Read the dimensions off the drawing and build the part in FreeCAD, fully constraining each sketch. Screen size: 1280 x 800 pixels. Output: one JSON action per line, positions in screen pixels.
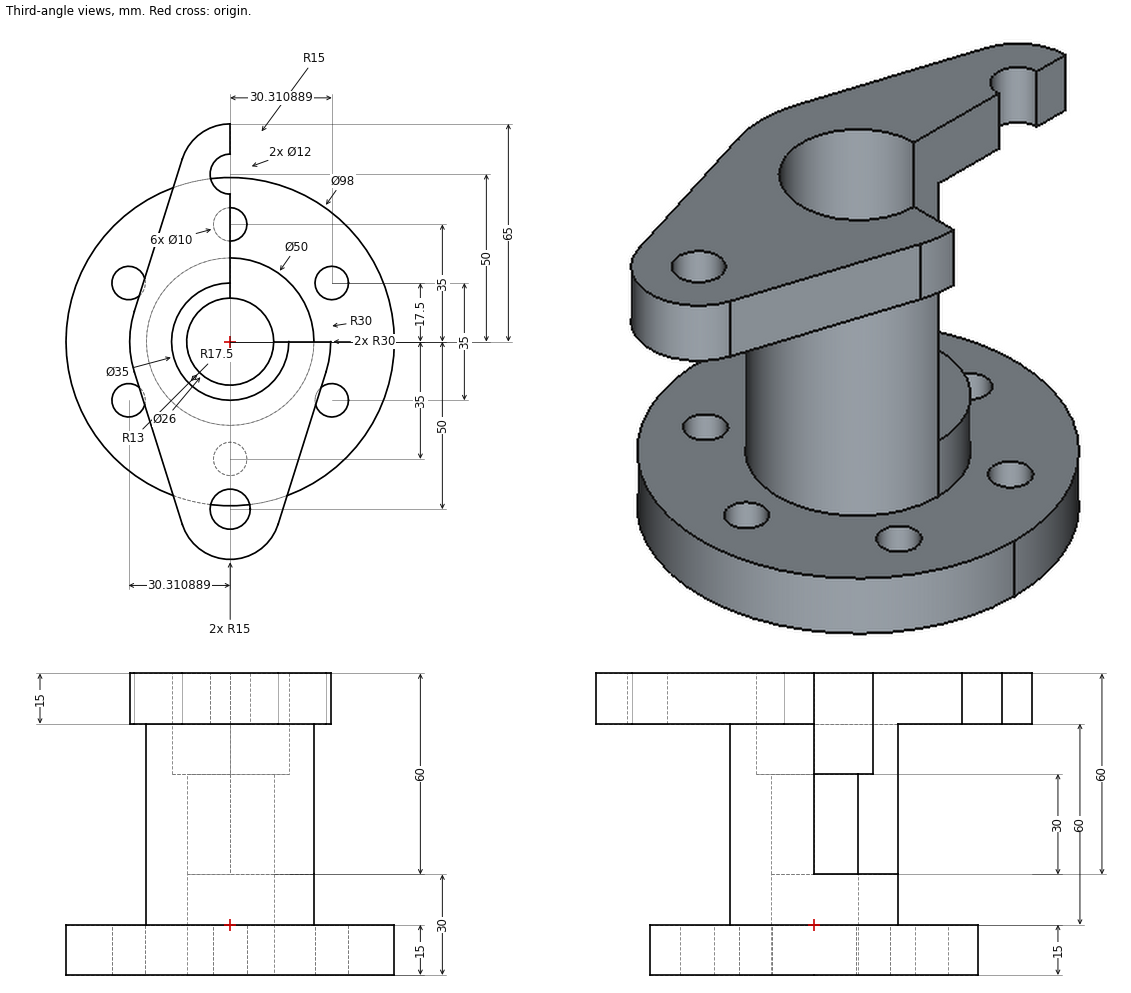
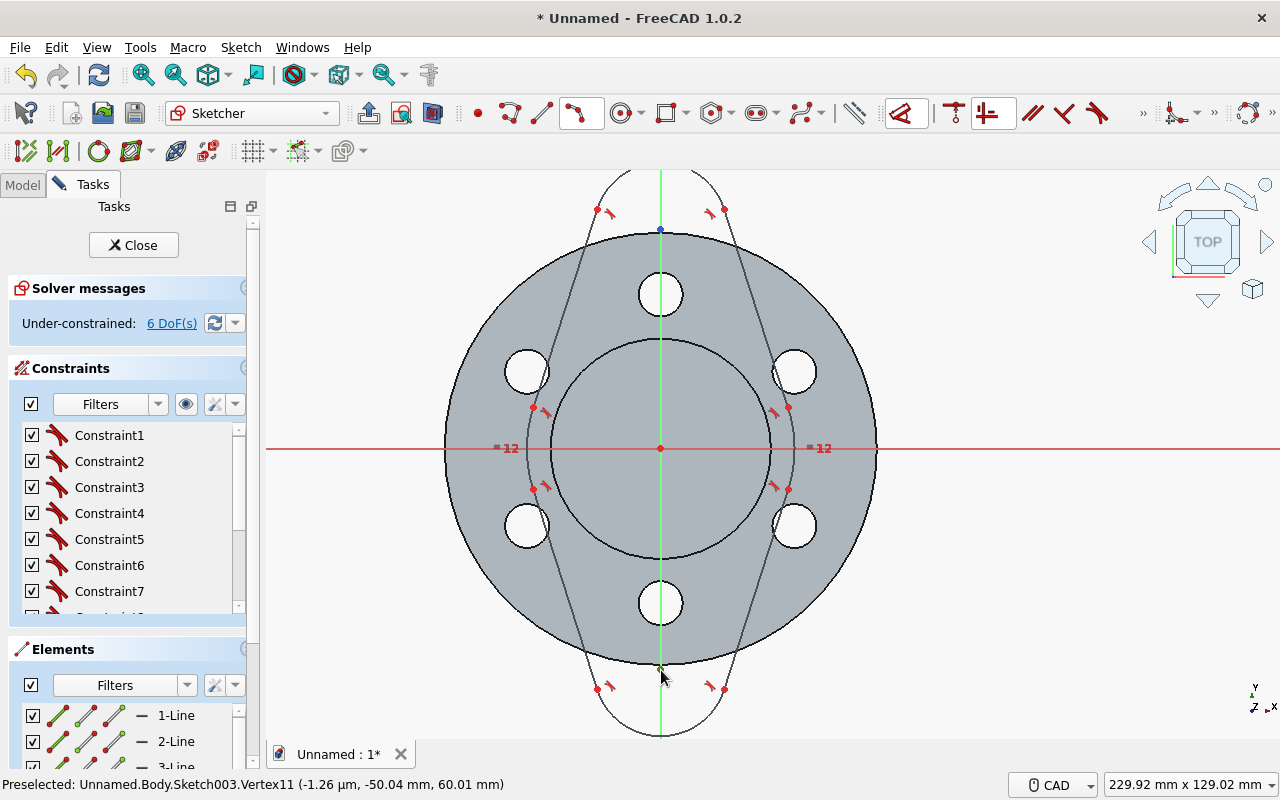
{"action": "left_click", "coordinate": [661, 674]}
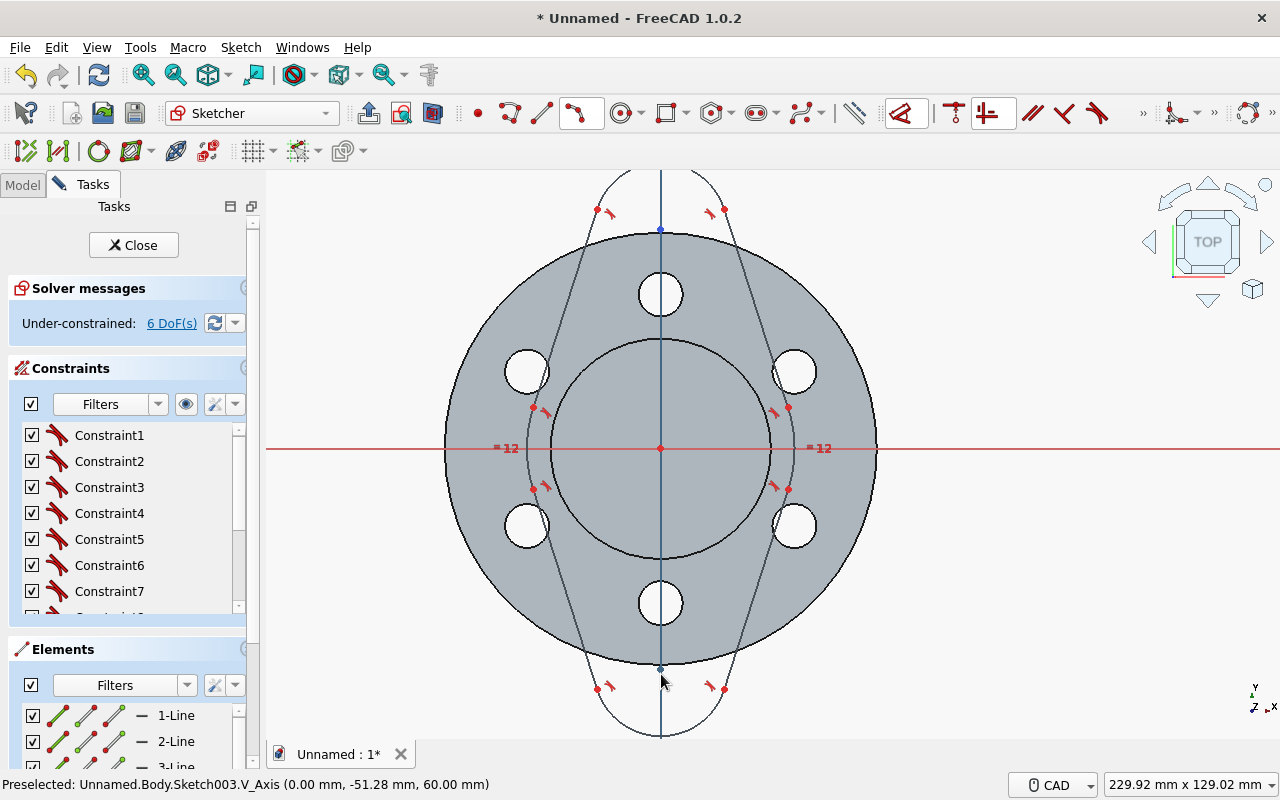
{"action": "left_click", "coordinate": [954, 114]}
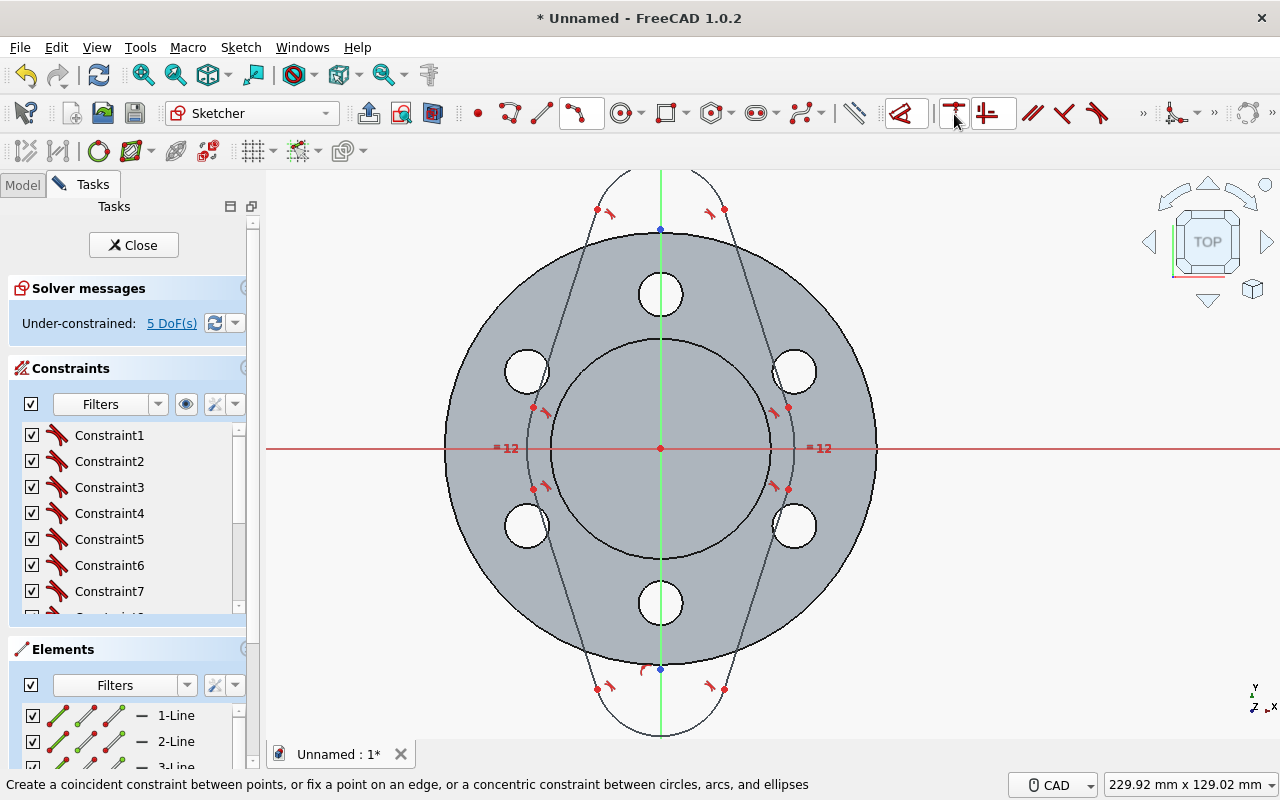
{"action": "left_click", "coordinate": [661, 230]}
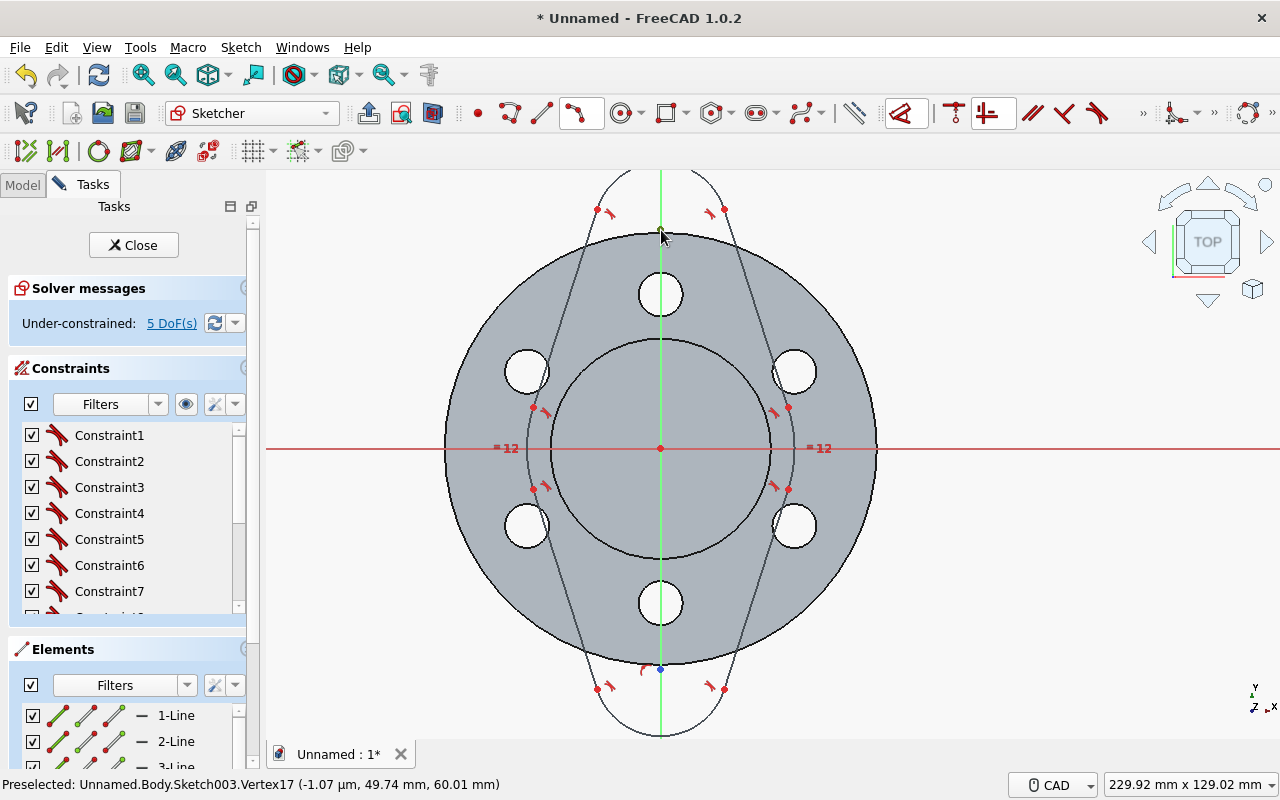
{"action": "left_click", "coordinate": [661, 674]}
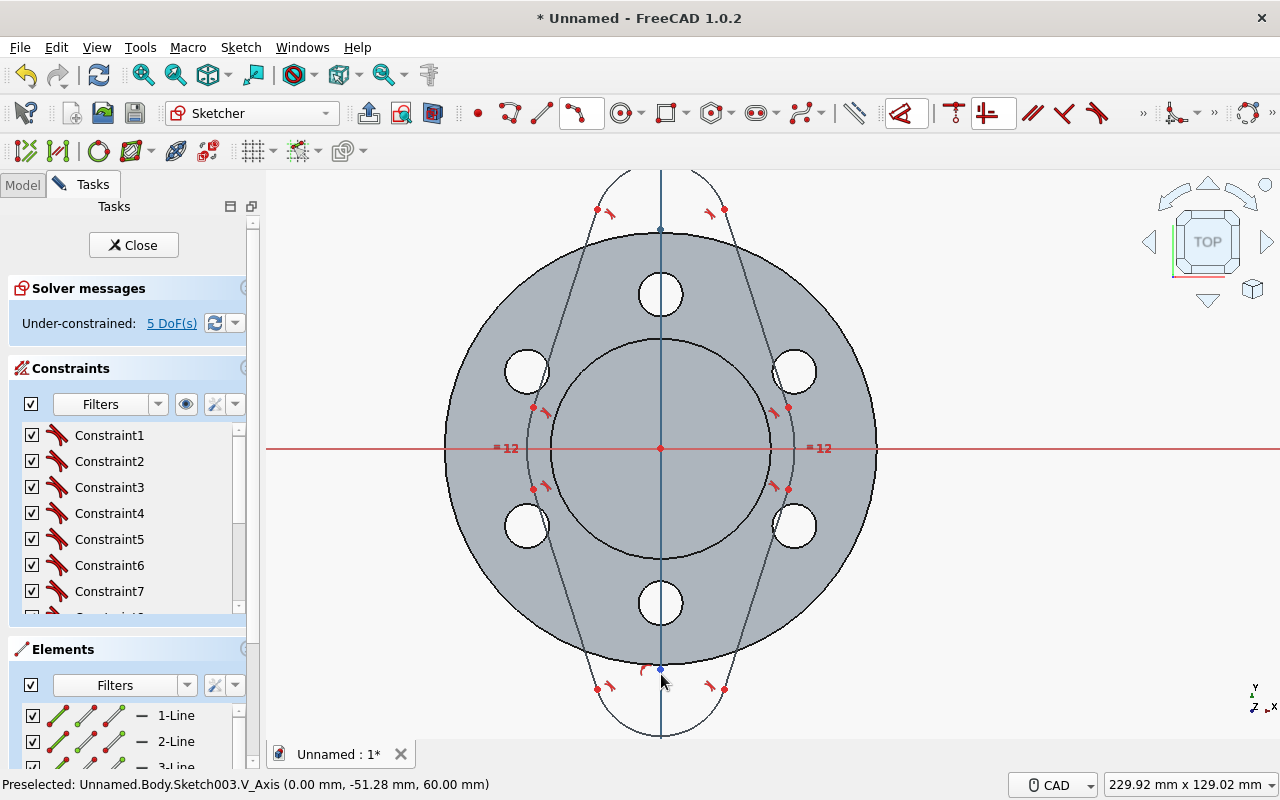
{"action": "left_click", "coordinate": [954, 114]}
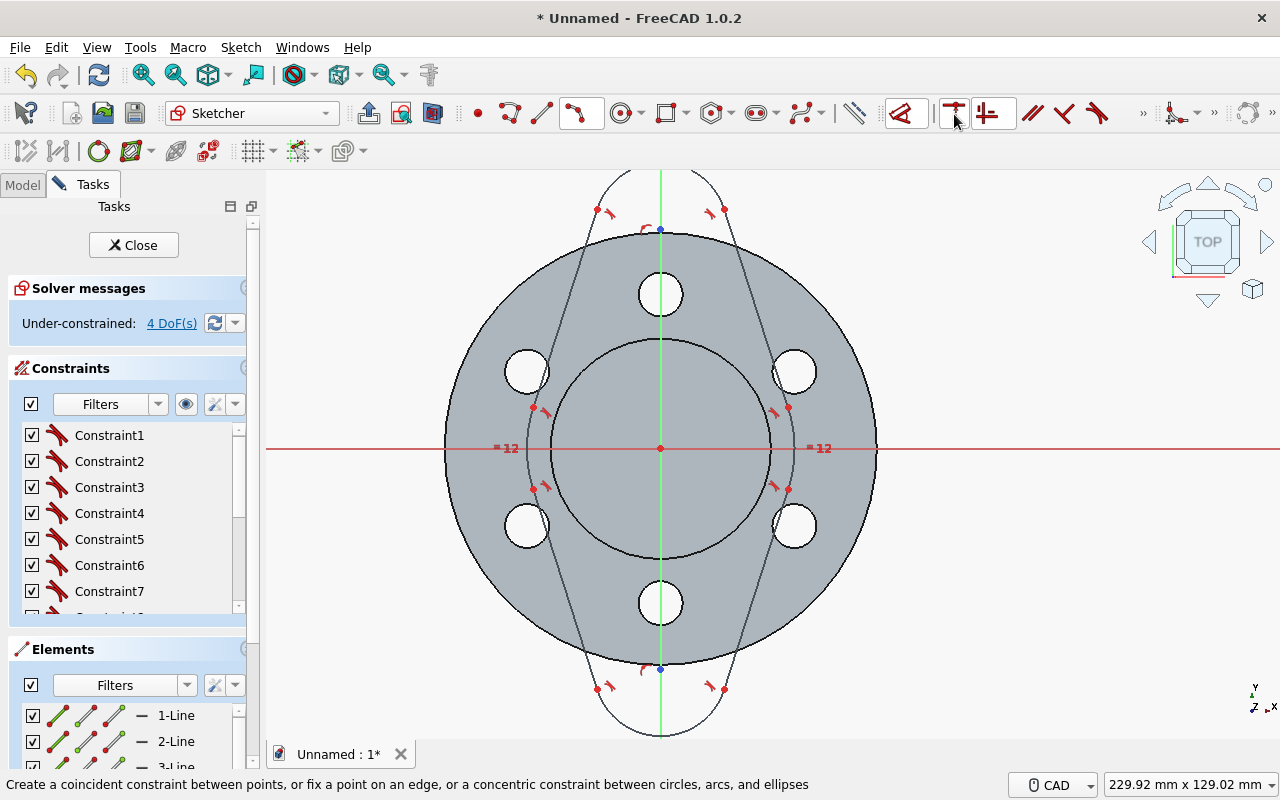
{"action": "scroll", "coordinate": [794, 466], "scroll_direction": "down", "scroll_amount": 2}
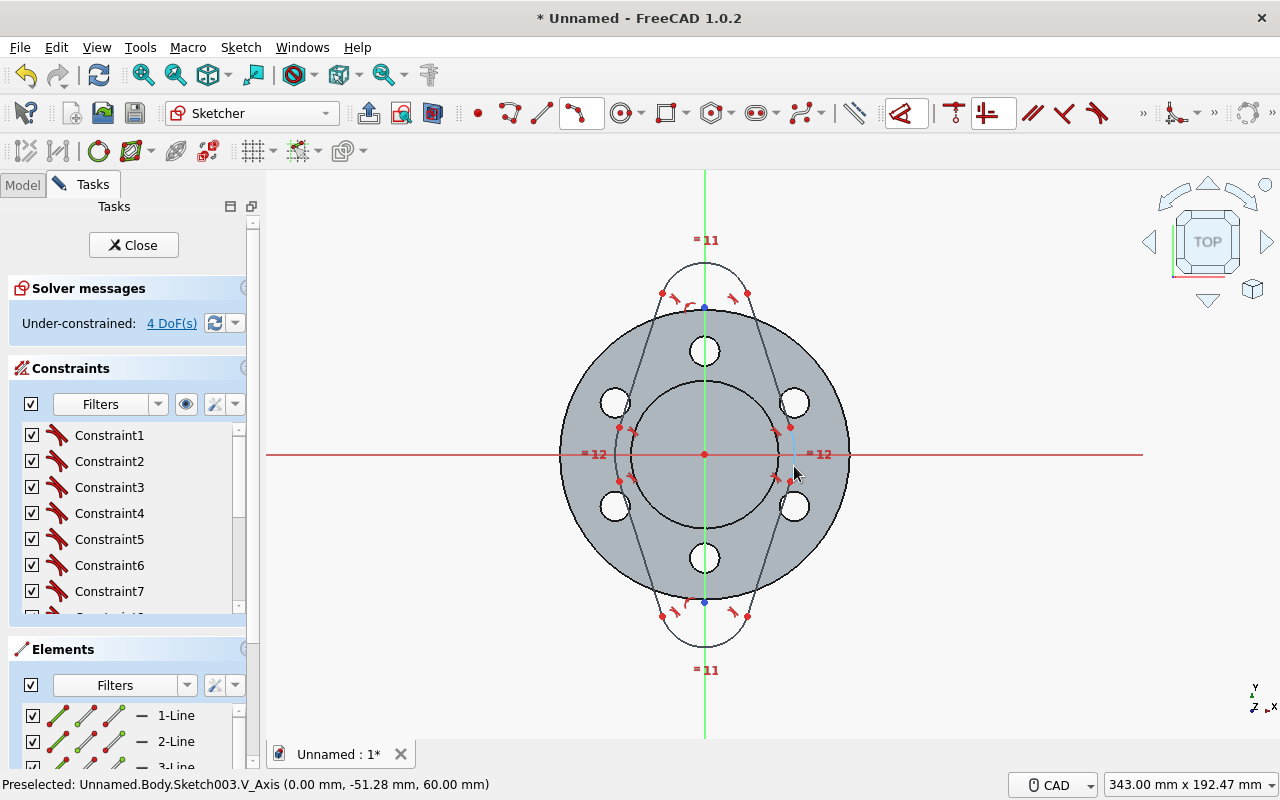
{"action": "left_click", "coordinate": [683, 642]}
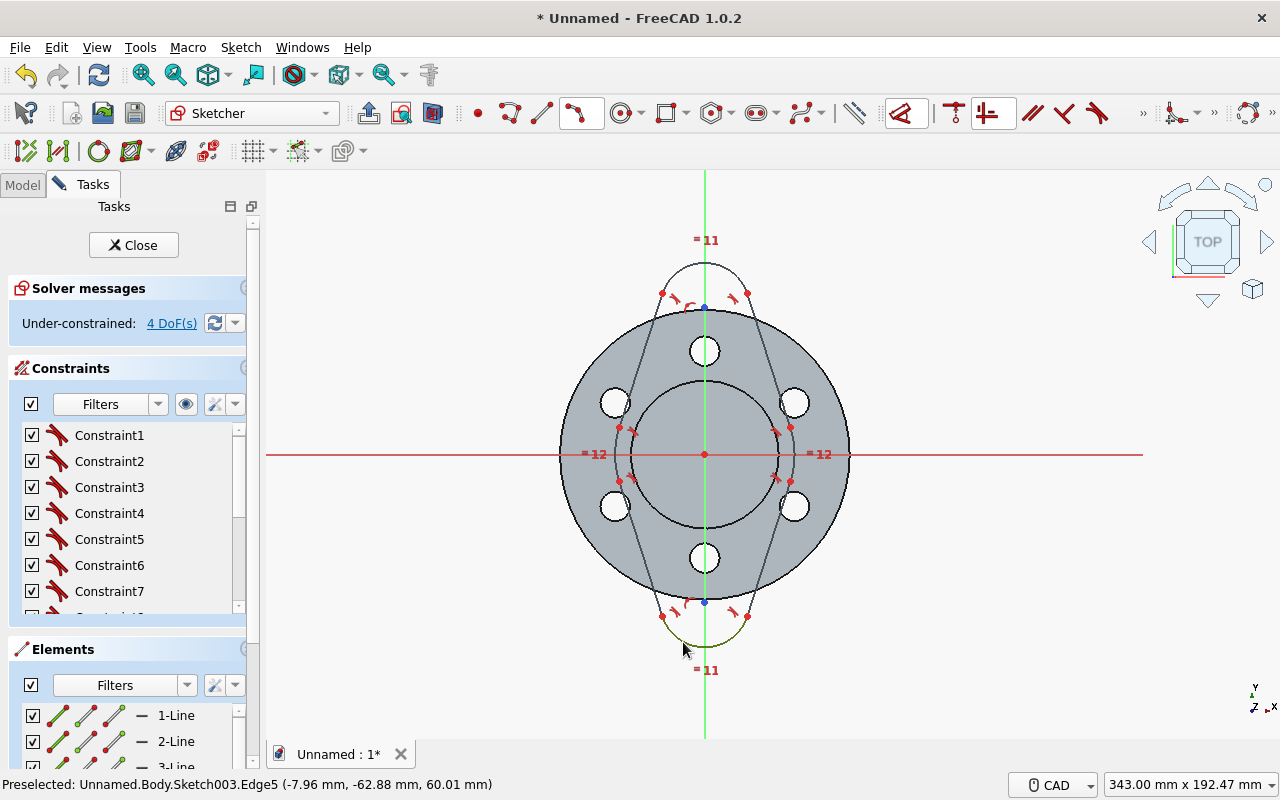
{"action": "key", "text": "k r"}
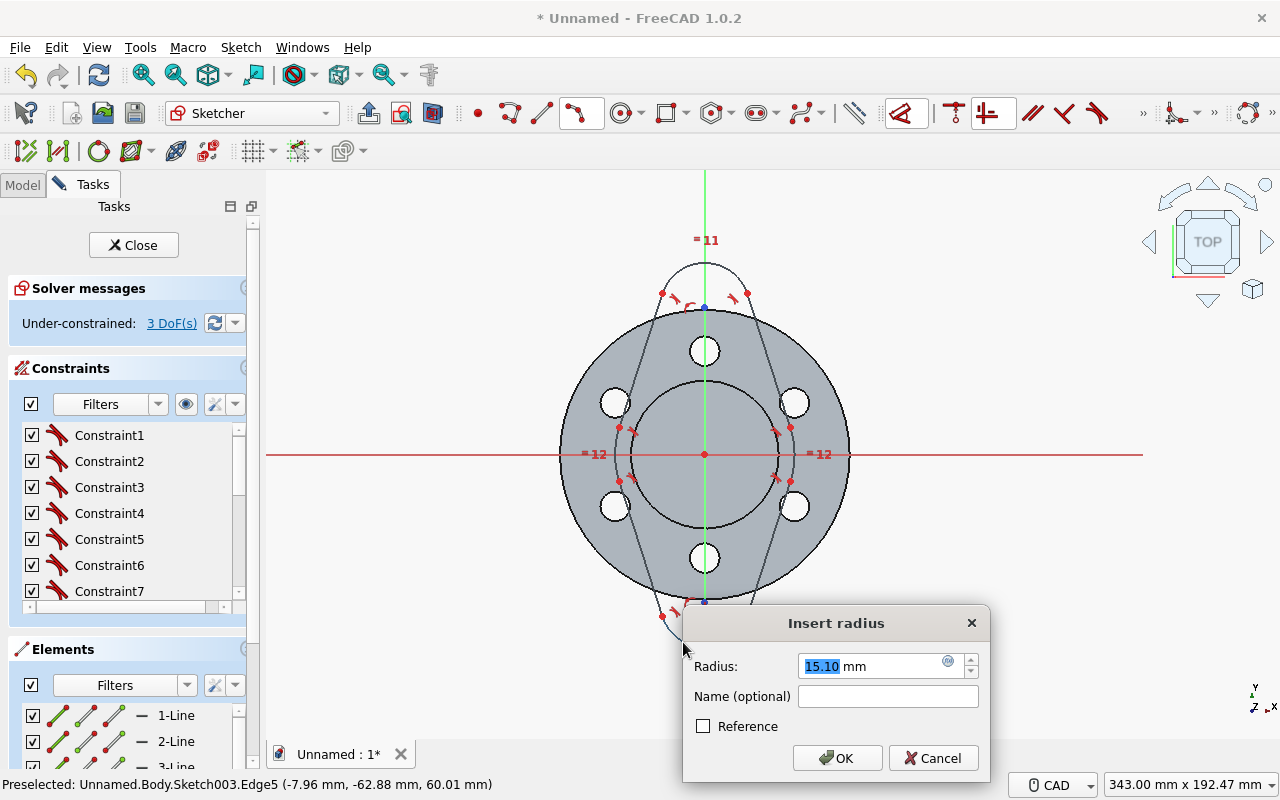
{"action": "type", "text": "15"}
{"action": "key", "text": "Return"}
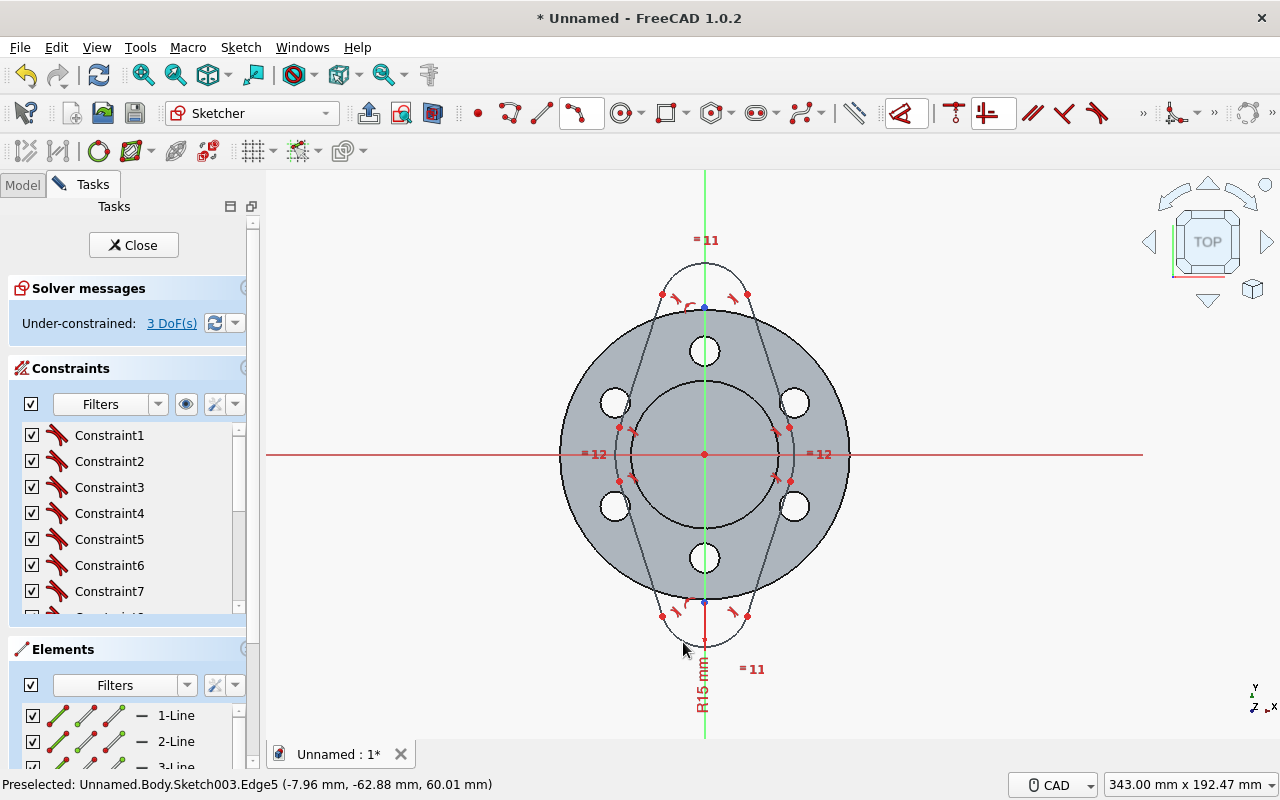
{"action": "scroll", "coordinate": [794, 466], "scroll_direction": "up", "scroll_amount": 2}